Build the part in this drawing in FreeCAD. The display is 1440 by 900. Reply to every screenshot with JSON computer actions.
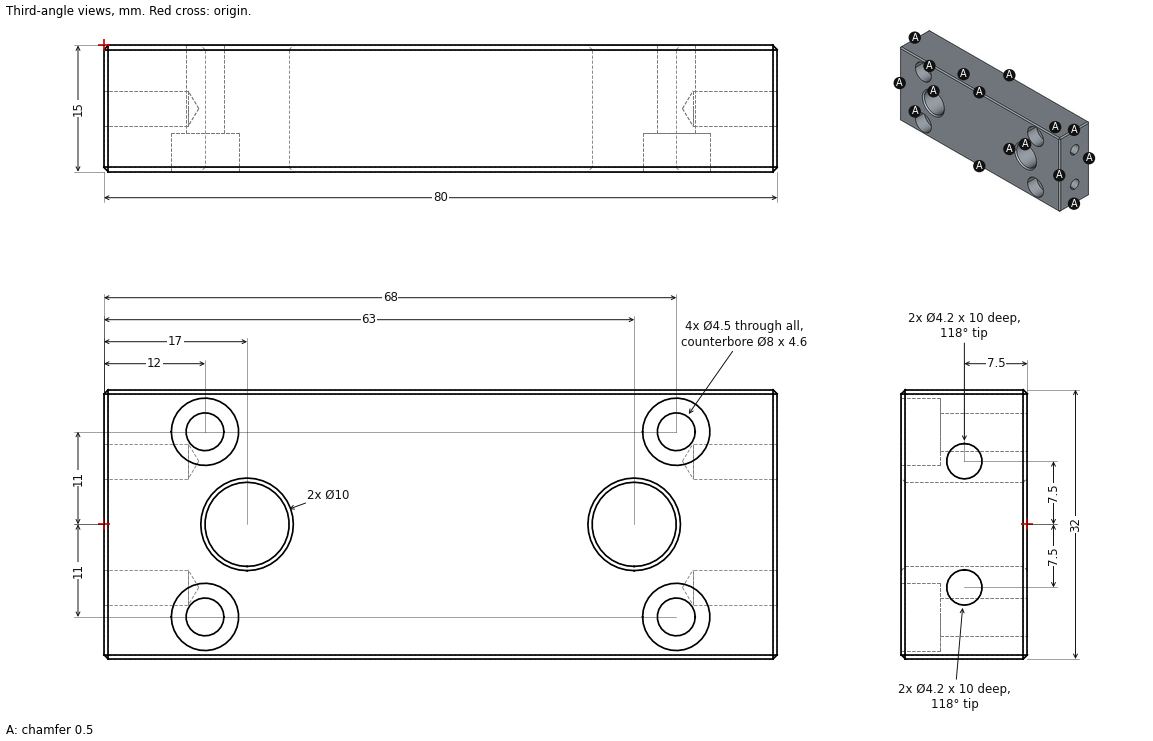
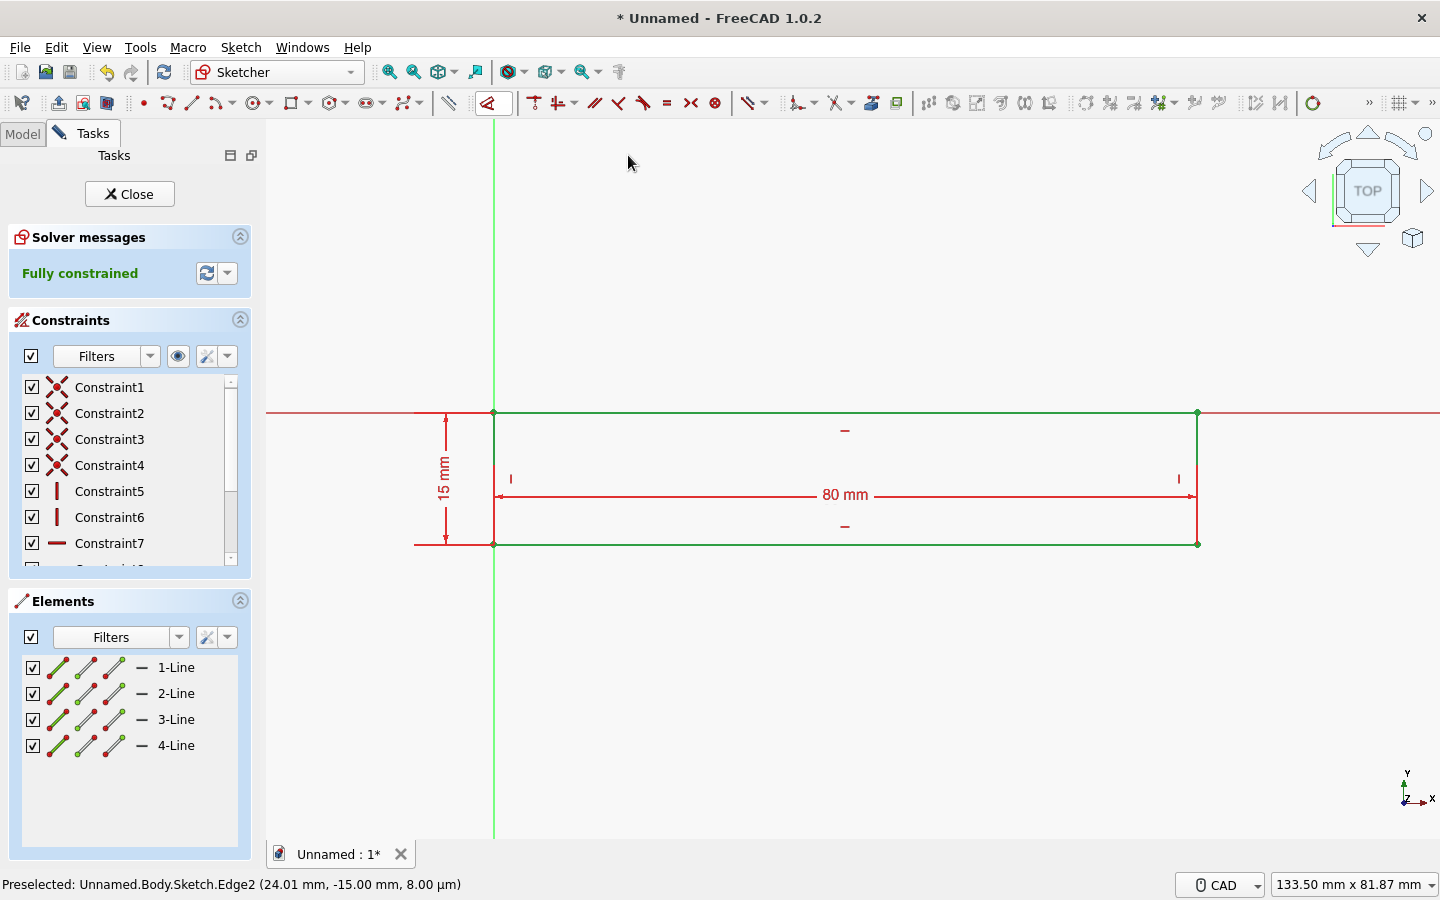
{"action": "left_click", "coordinate": [130, 194]}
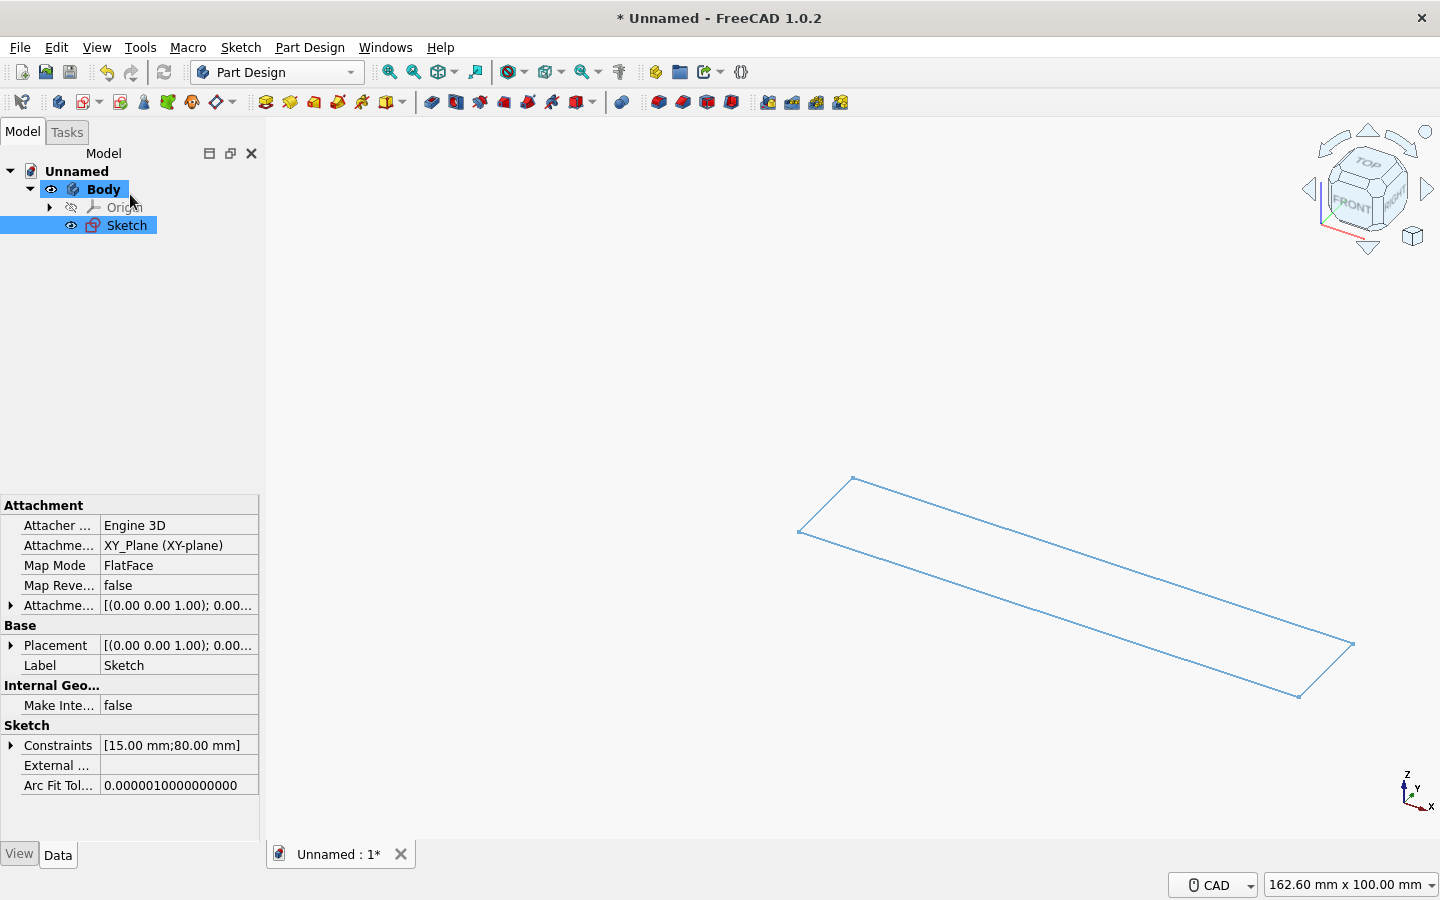
{"action": "left_click", "coordinate": [266, 102]}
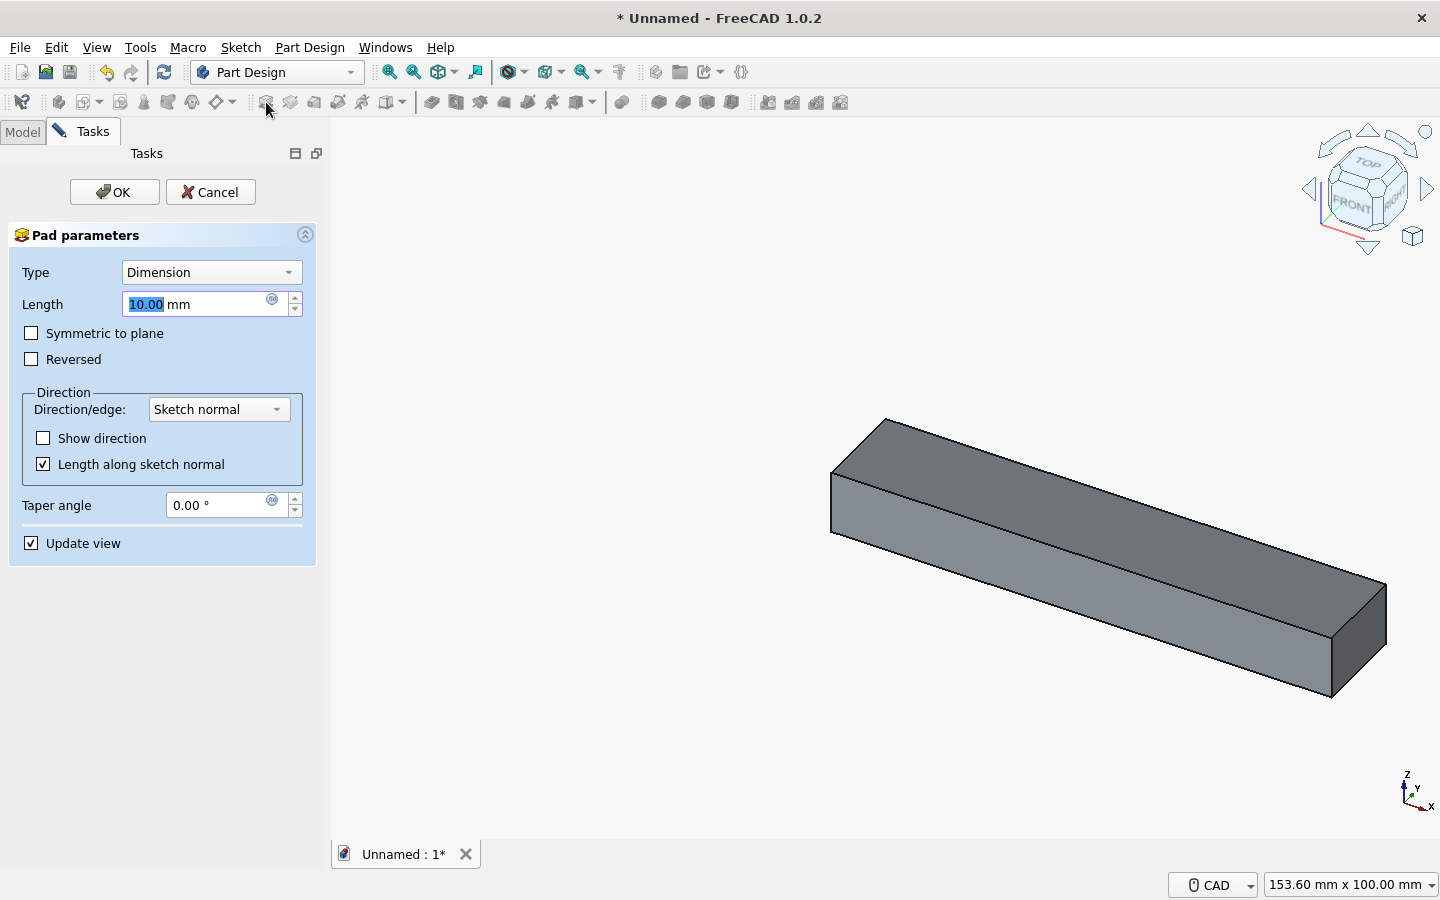
{"action": "type", "text": "32"}
{"action": "key", "text": "Tab"}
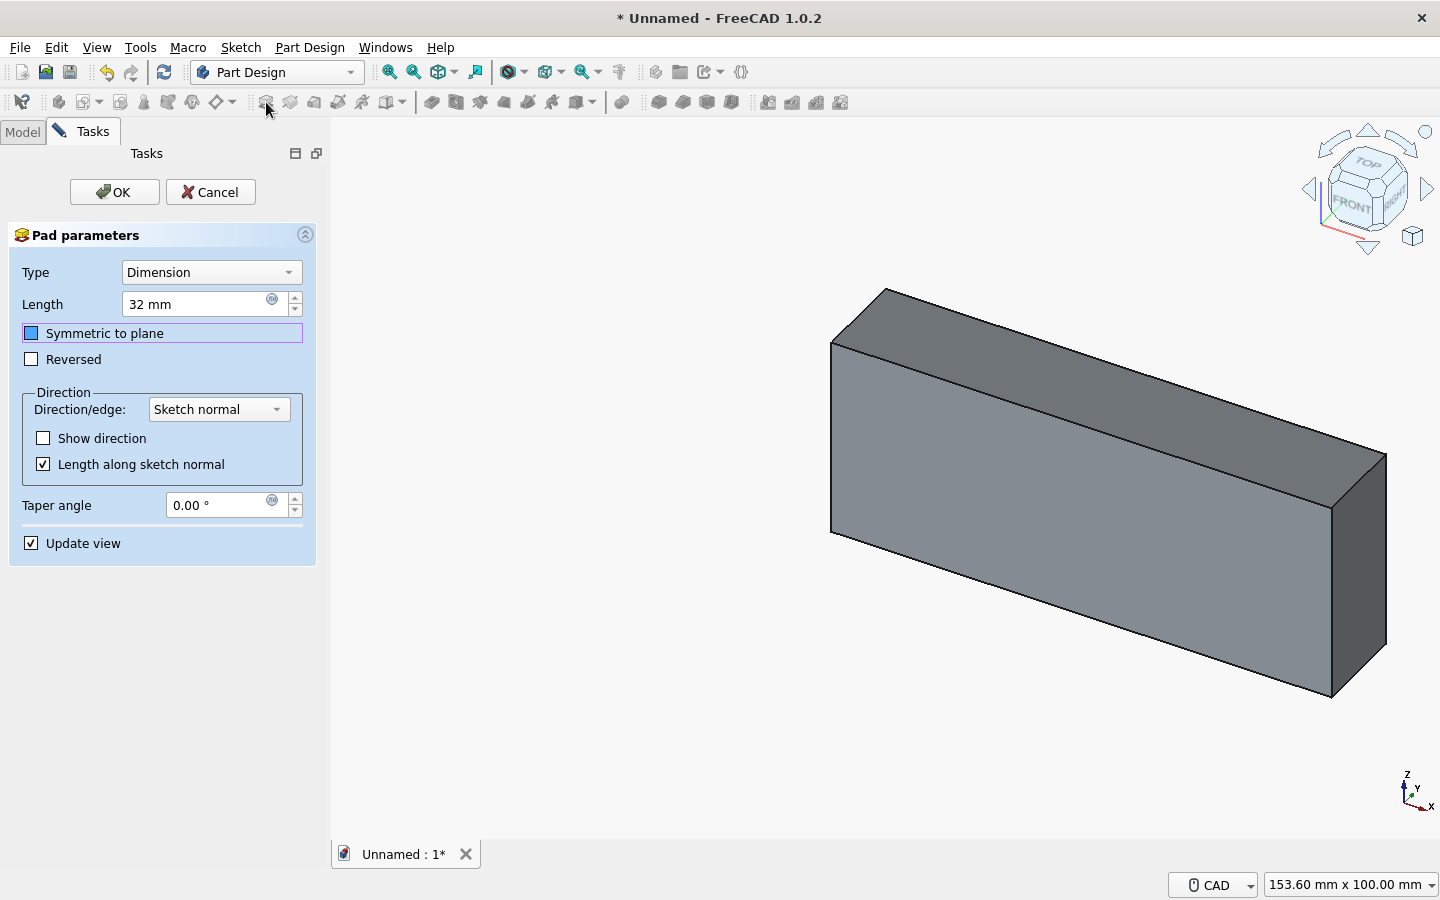
{"action": "left_click", "coordinate": [30, 333]}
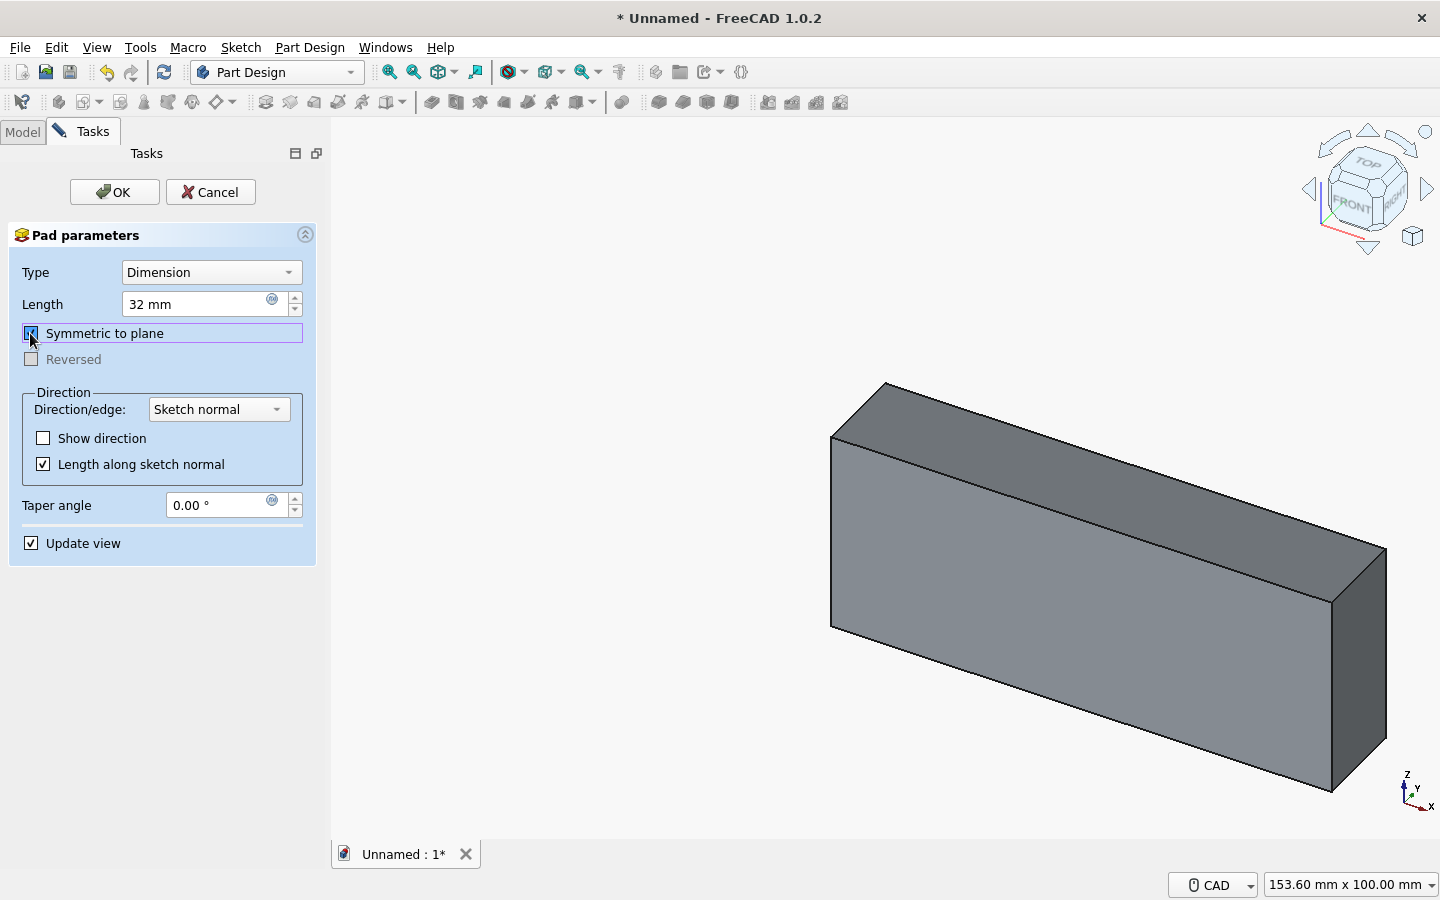
{"action": "left_click", "coordinate": [115, 192]}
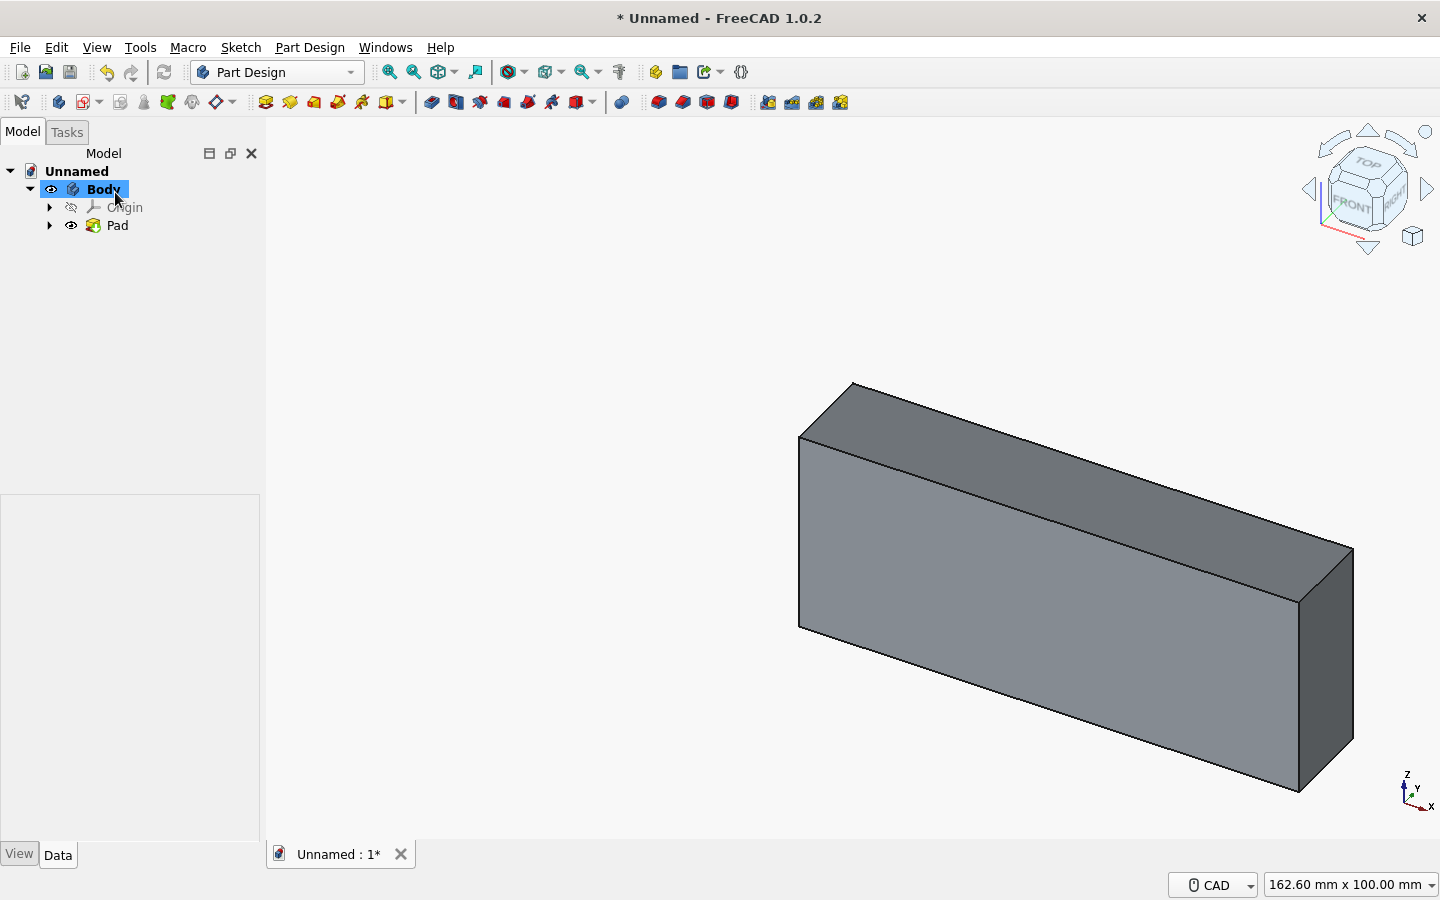
{"action": "left_click", "coordinate": [1192, 661]}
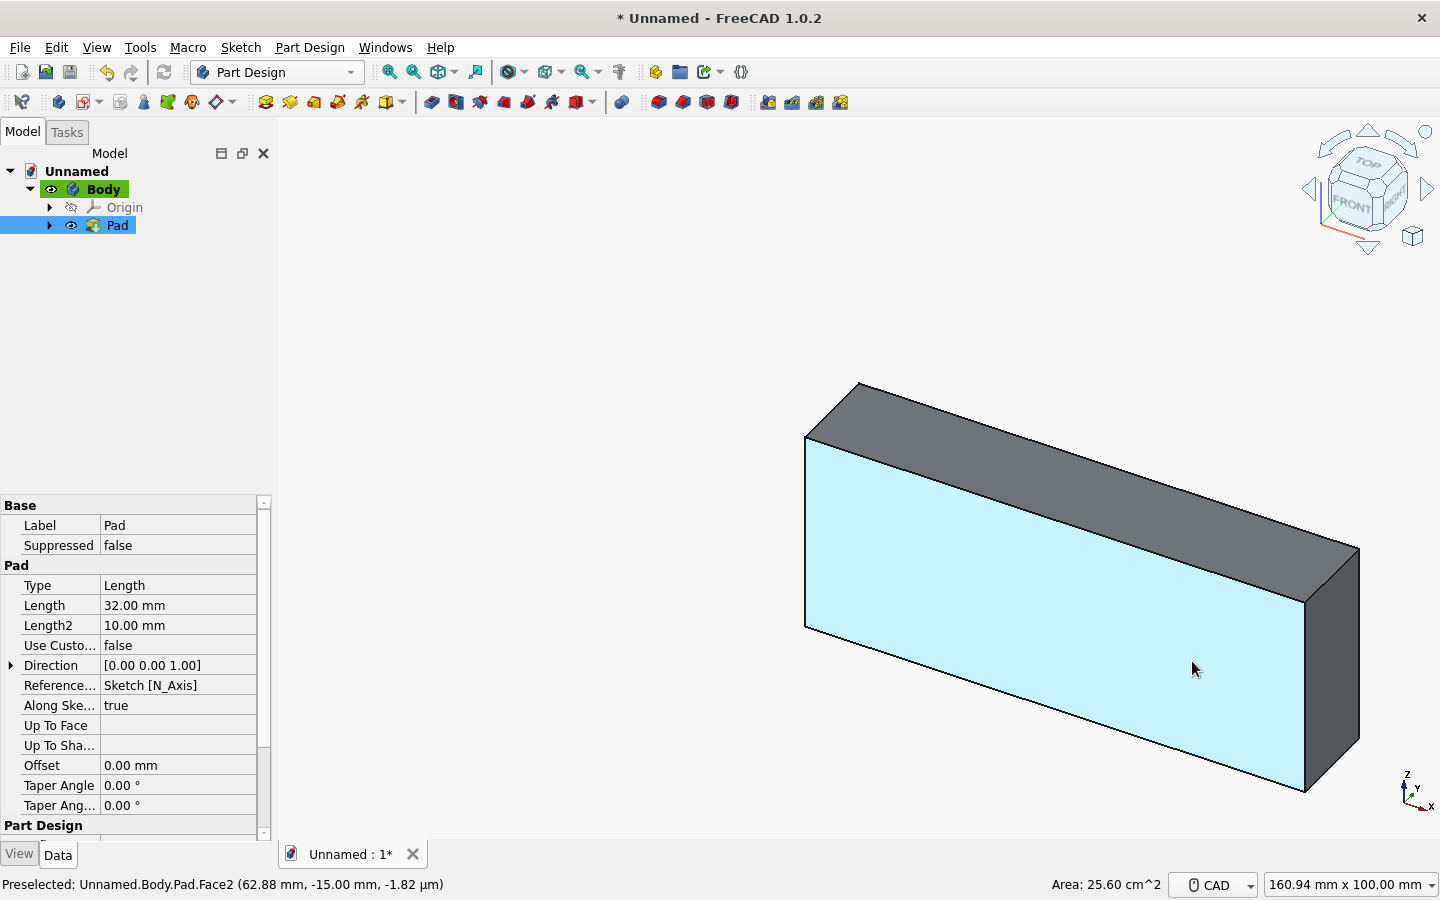
{"action": "left_click", "coordinate": [84, 102]}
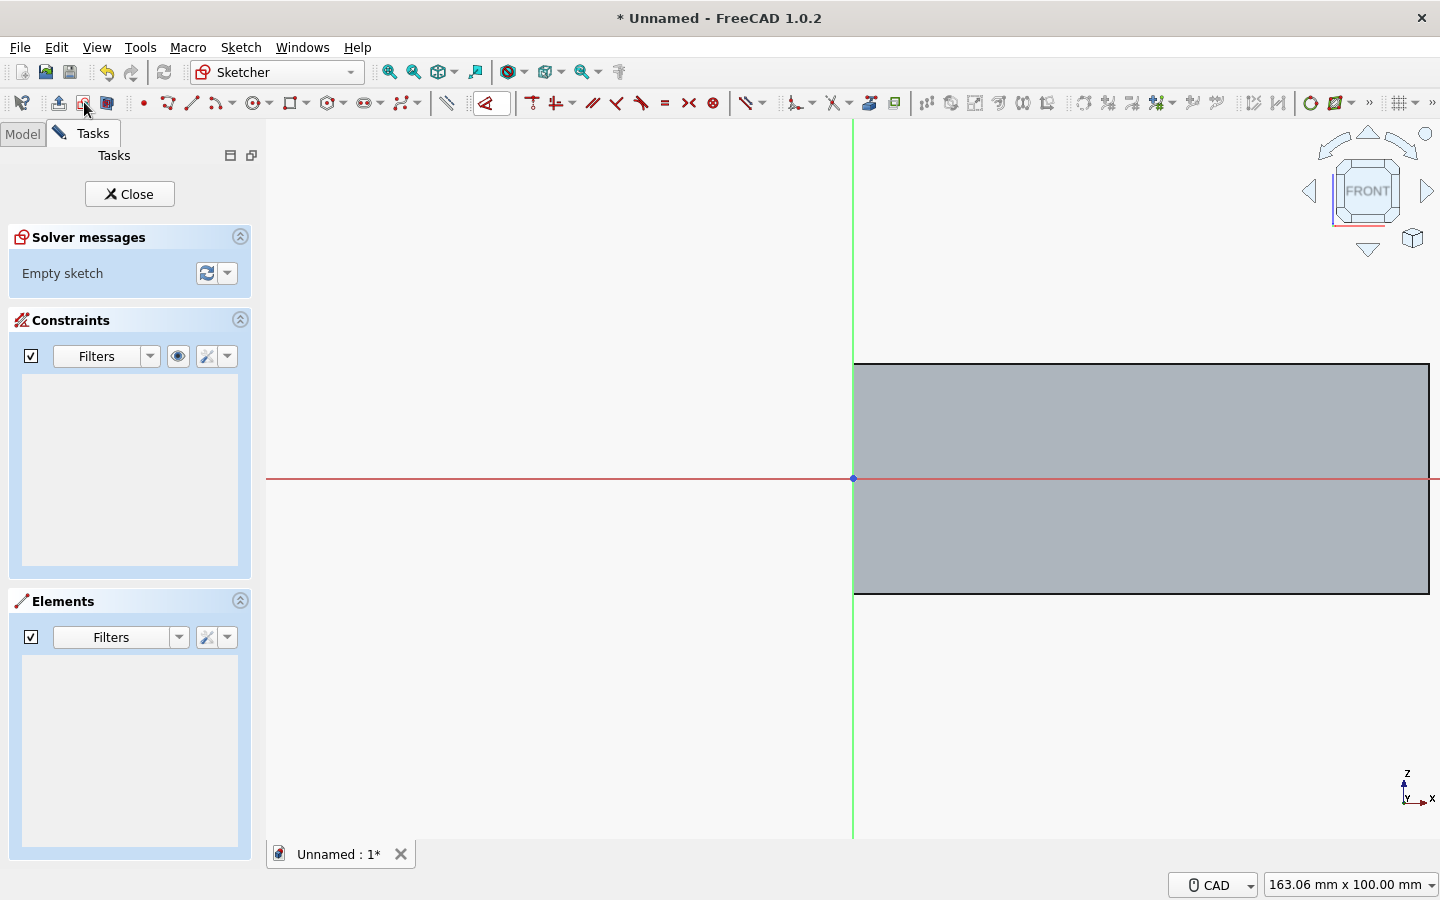
{"action": "scroll", "coordinate": [294, 479], "scroll_direction": "down", "scroll_amount": 1}